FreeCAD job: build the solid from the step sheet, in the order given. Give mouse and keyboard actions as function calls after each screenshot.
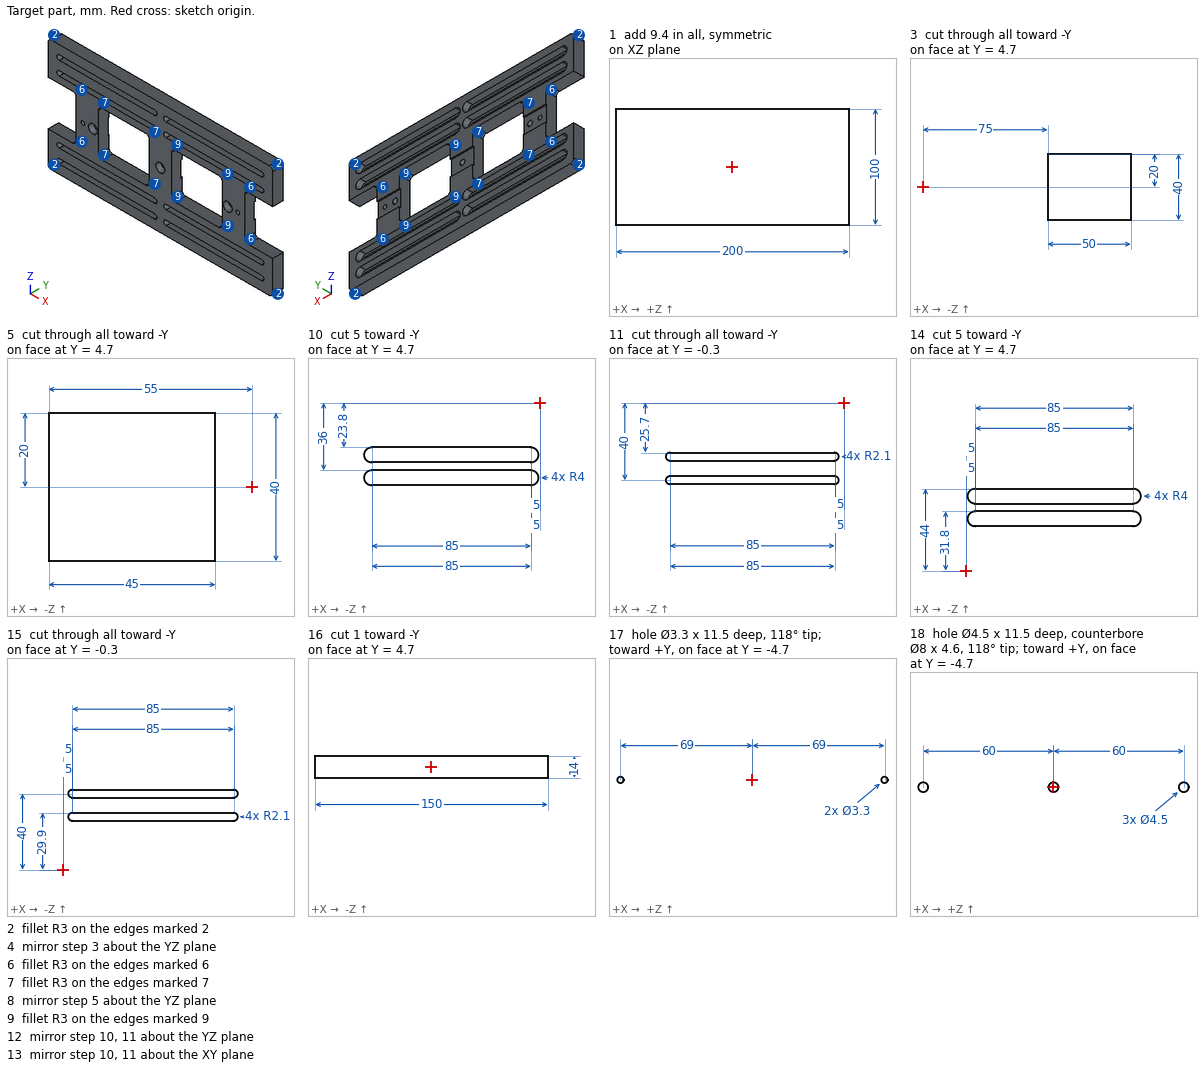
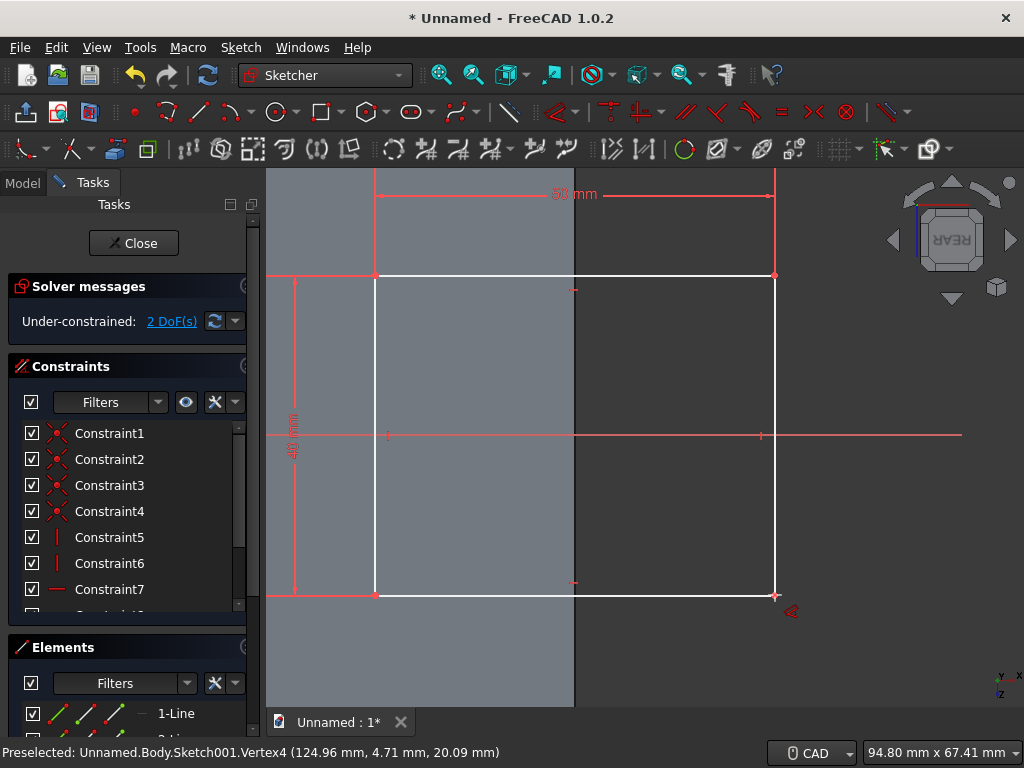
click(375, 276)
click(335, 242)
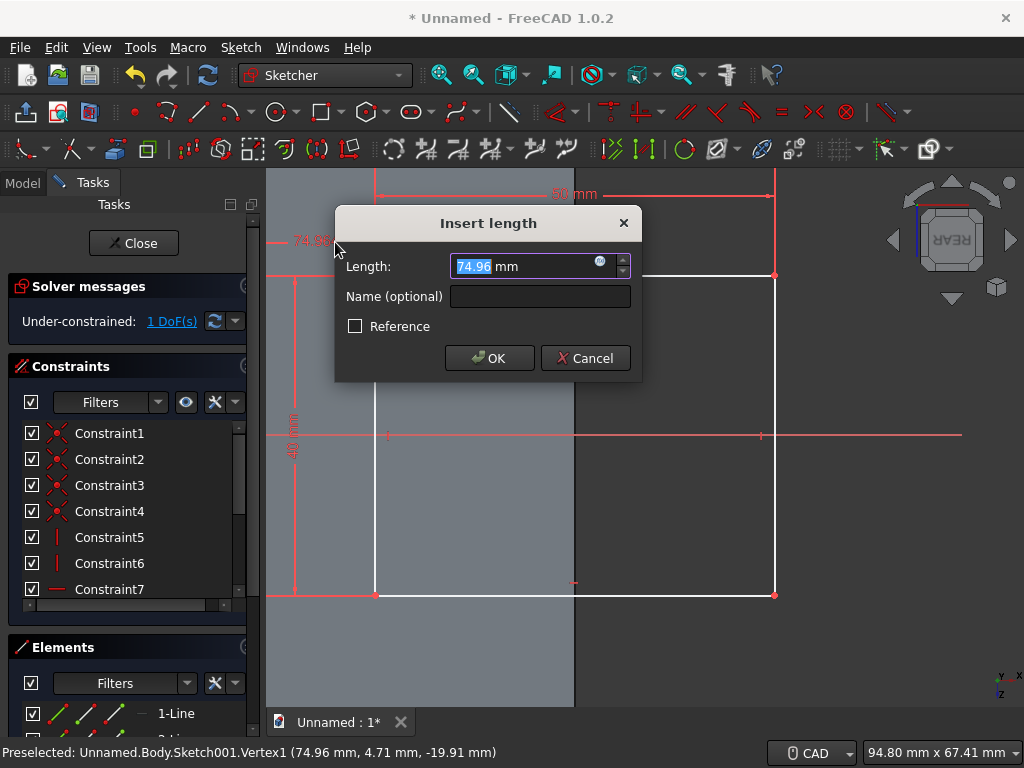
text(75)
key(Return)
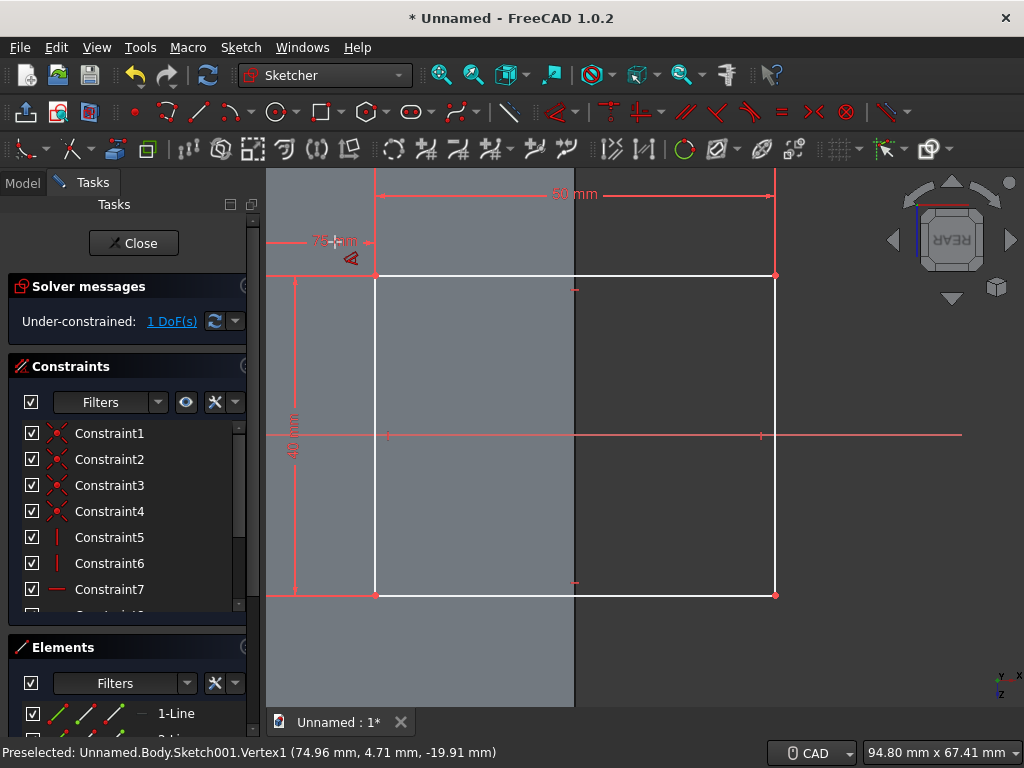
click(375, 276)
click(409, 356)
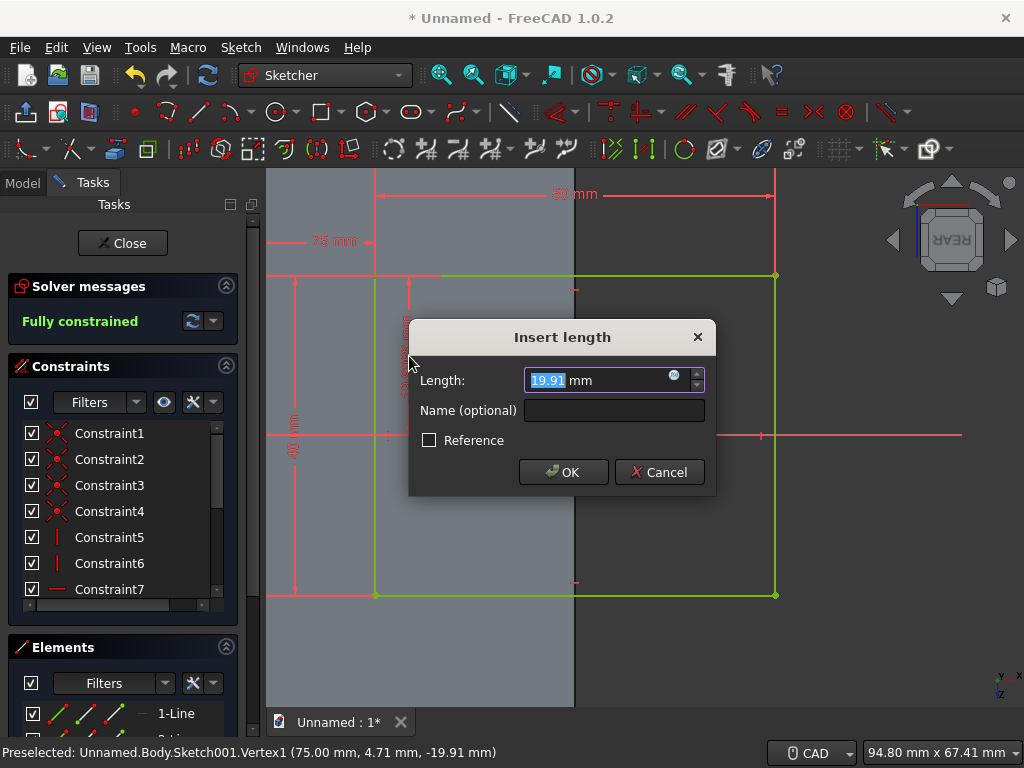
text(20)
key(Return)
key(Escape)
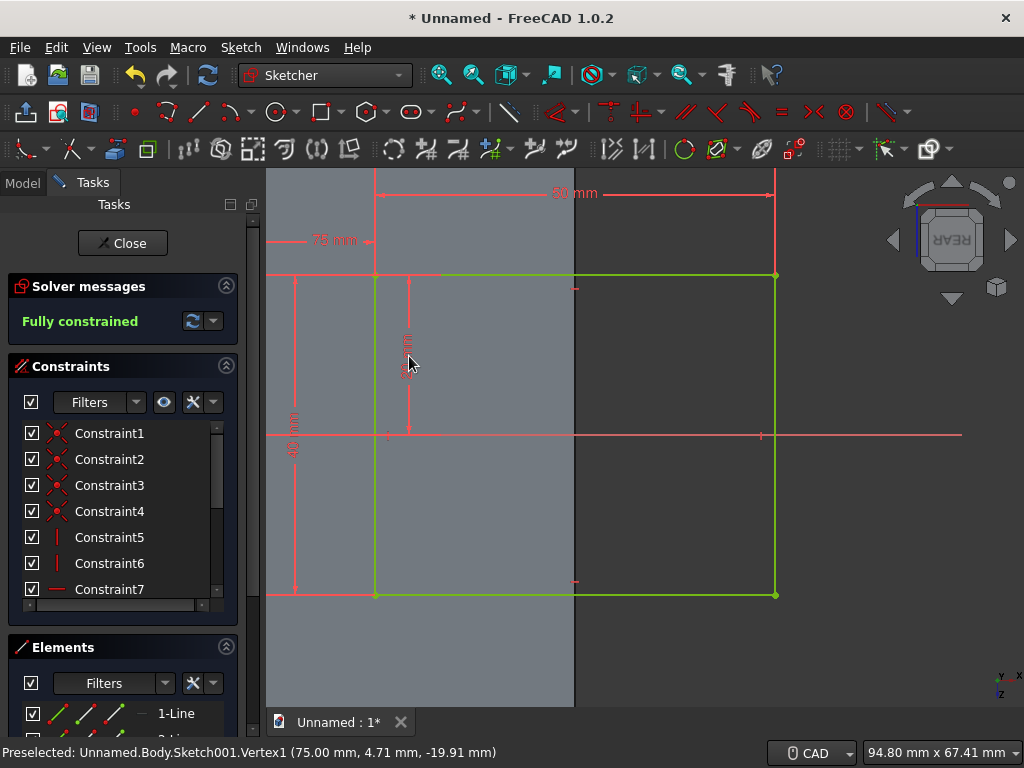
click(123, 243)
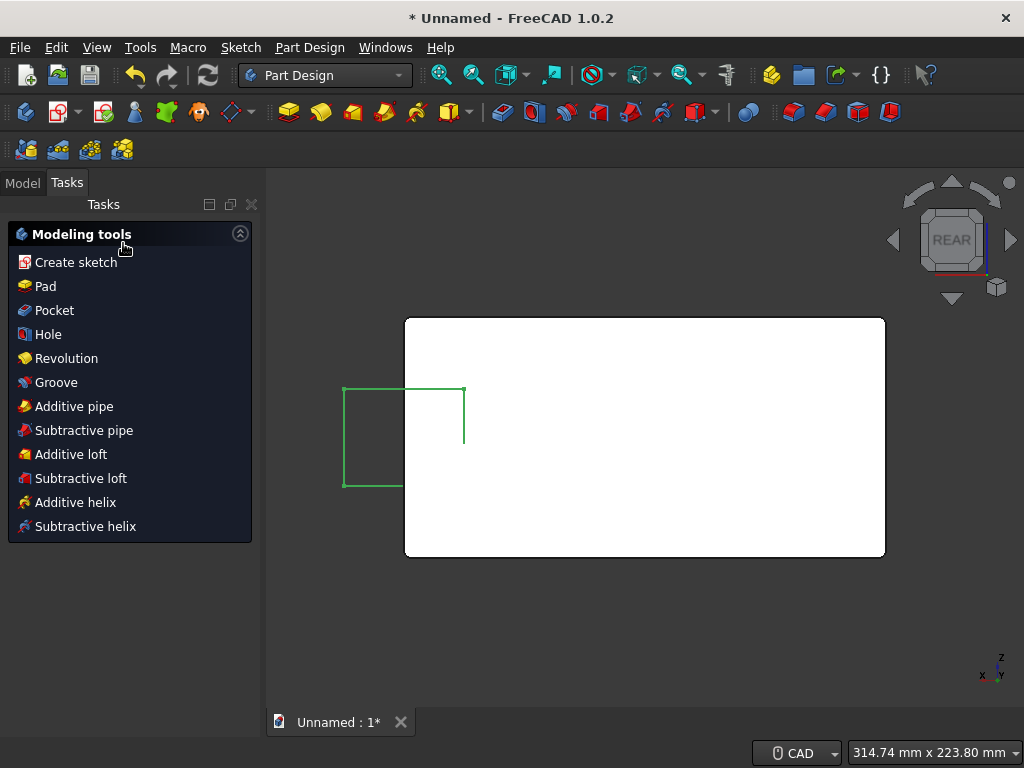
click(504, 112)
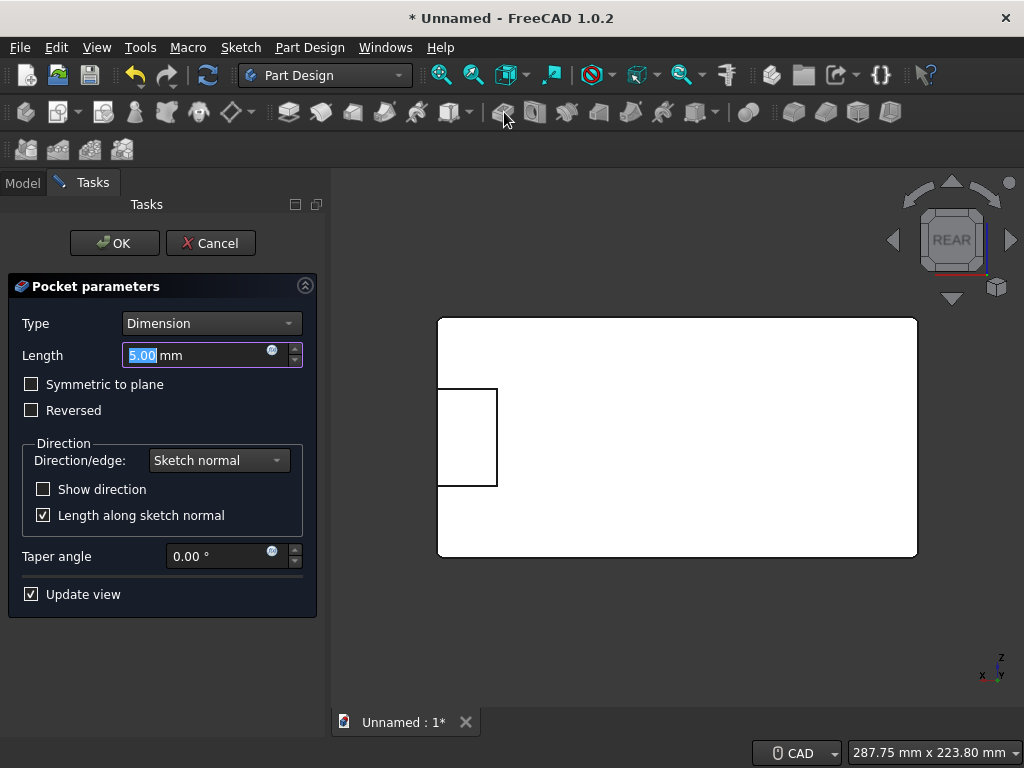
click(212, 324)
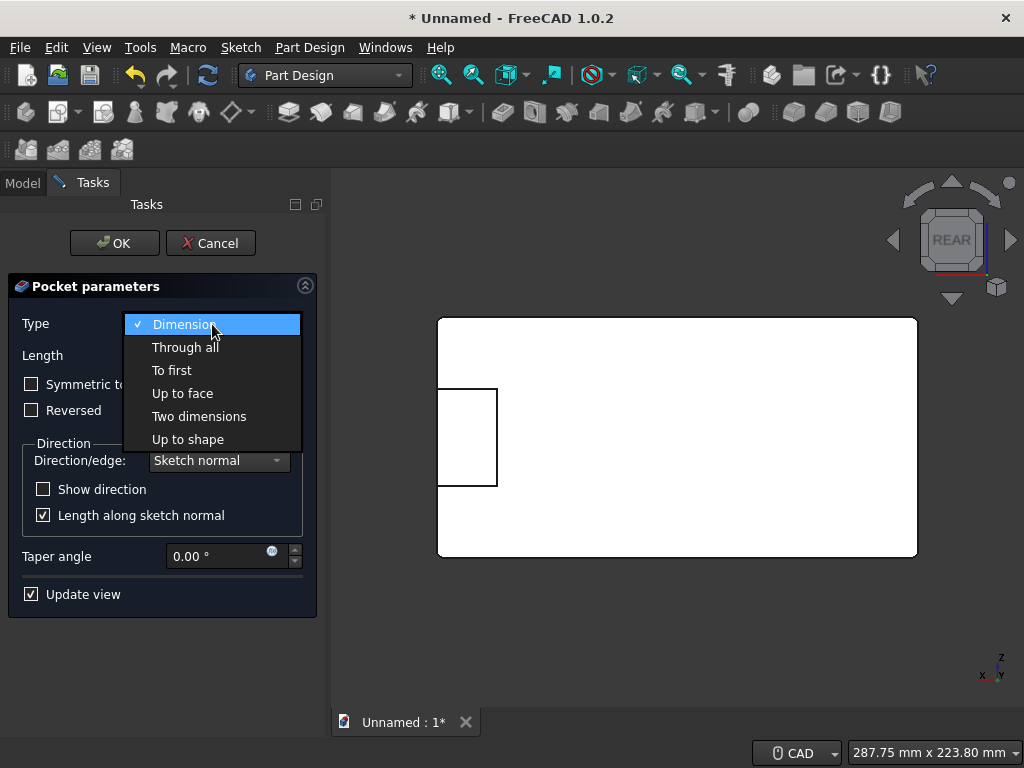
click(212, 348)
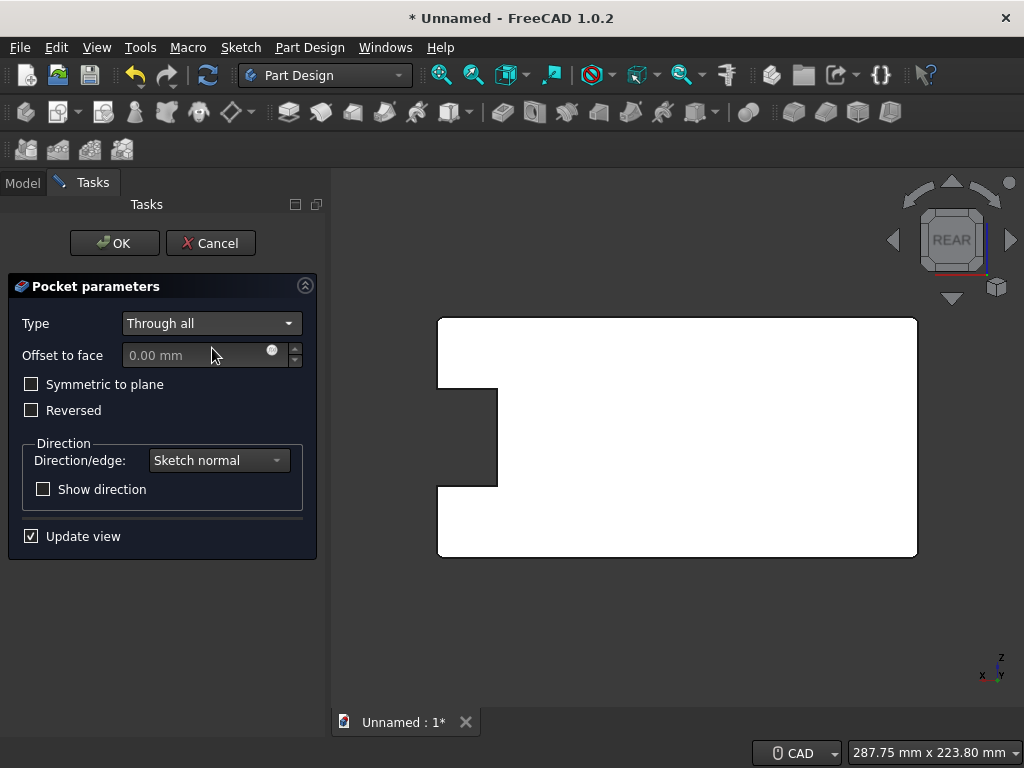
click(115, 243)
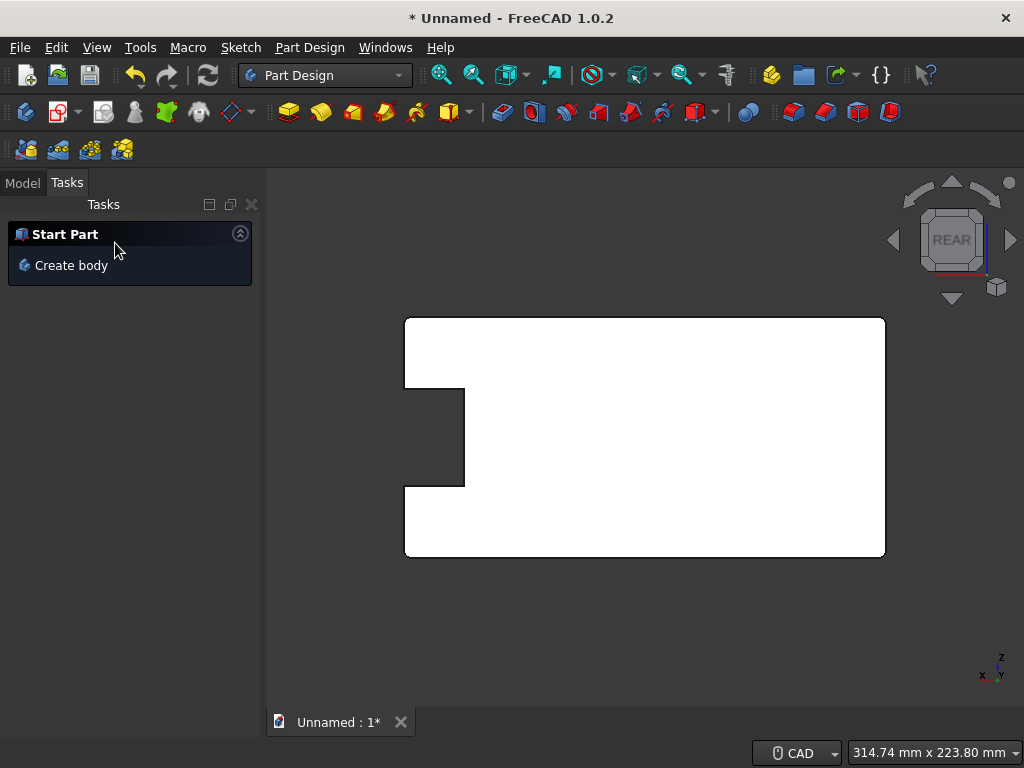
click(23, 182)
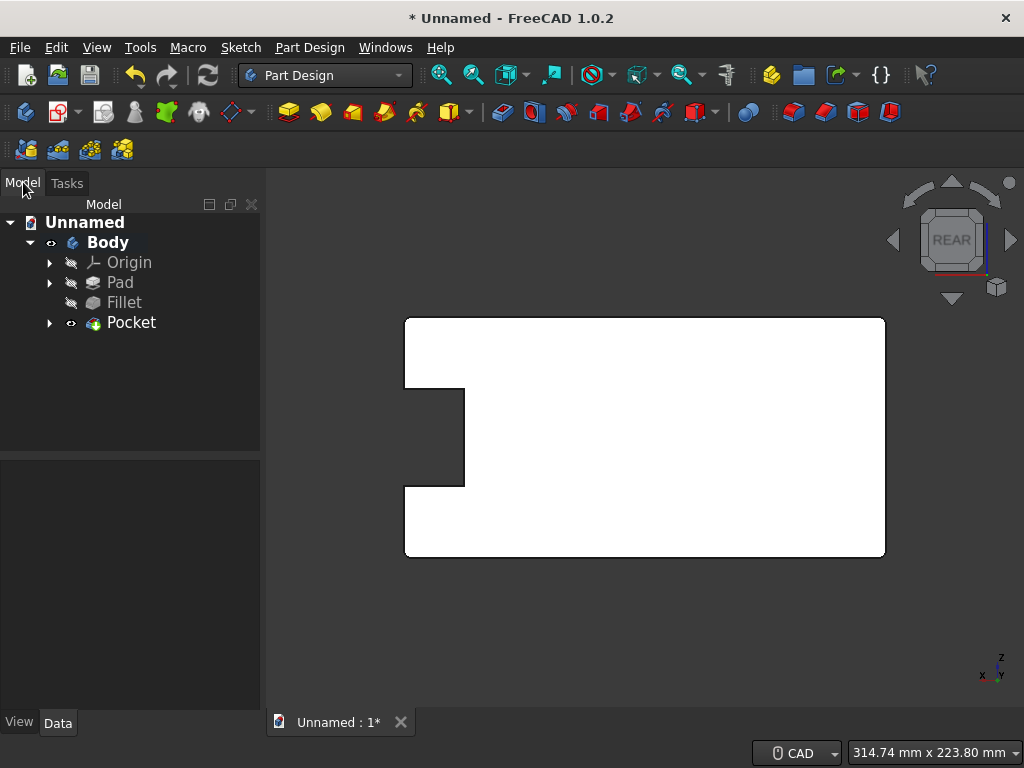
click(116, 323)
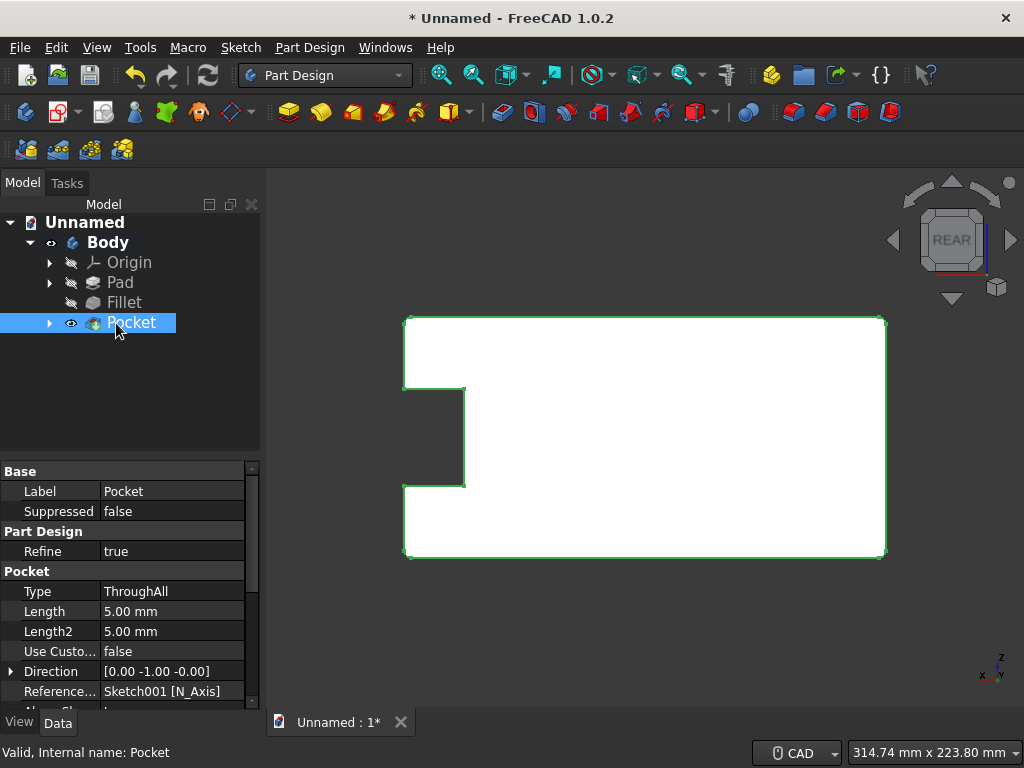
click(26, 150)